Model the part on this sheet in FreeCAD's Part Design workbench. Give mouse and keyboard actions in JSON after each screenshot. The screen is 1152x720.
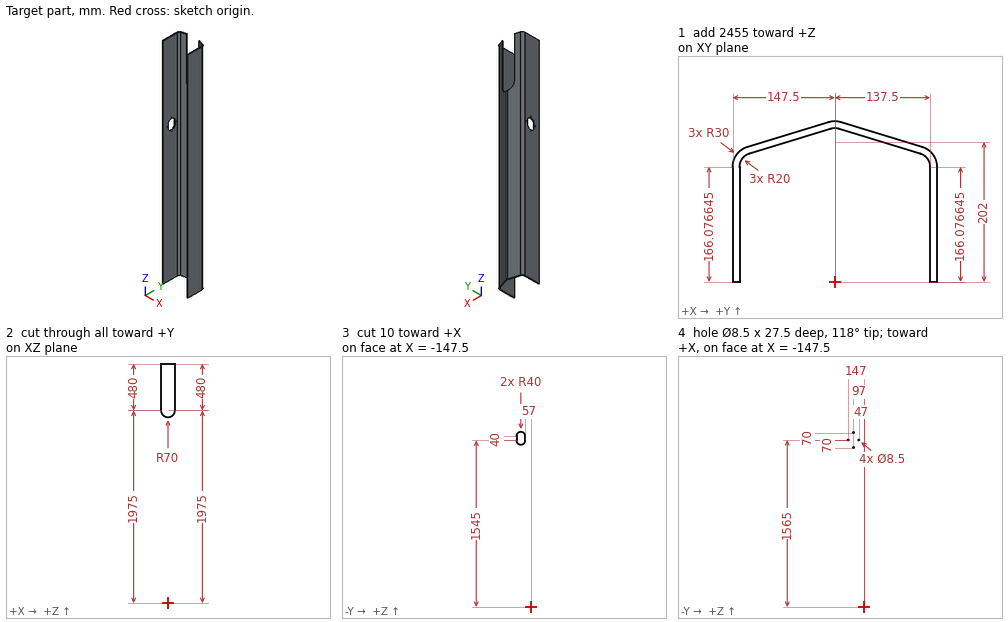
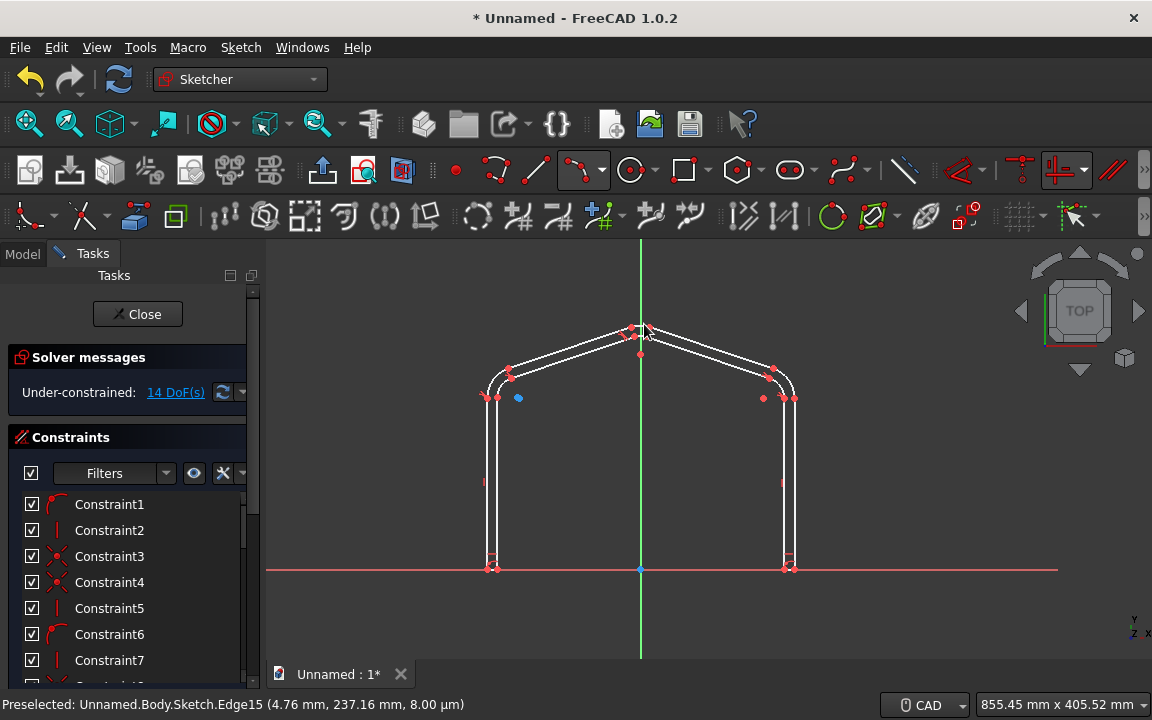
{"action": "scroll", "coordinate": [505, 382], "scroll_direction": "up", "scroll_amount": 3}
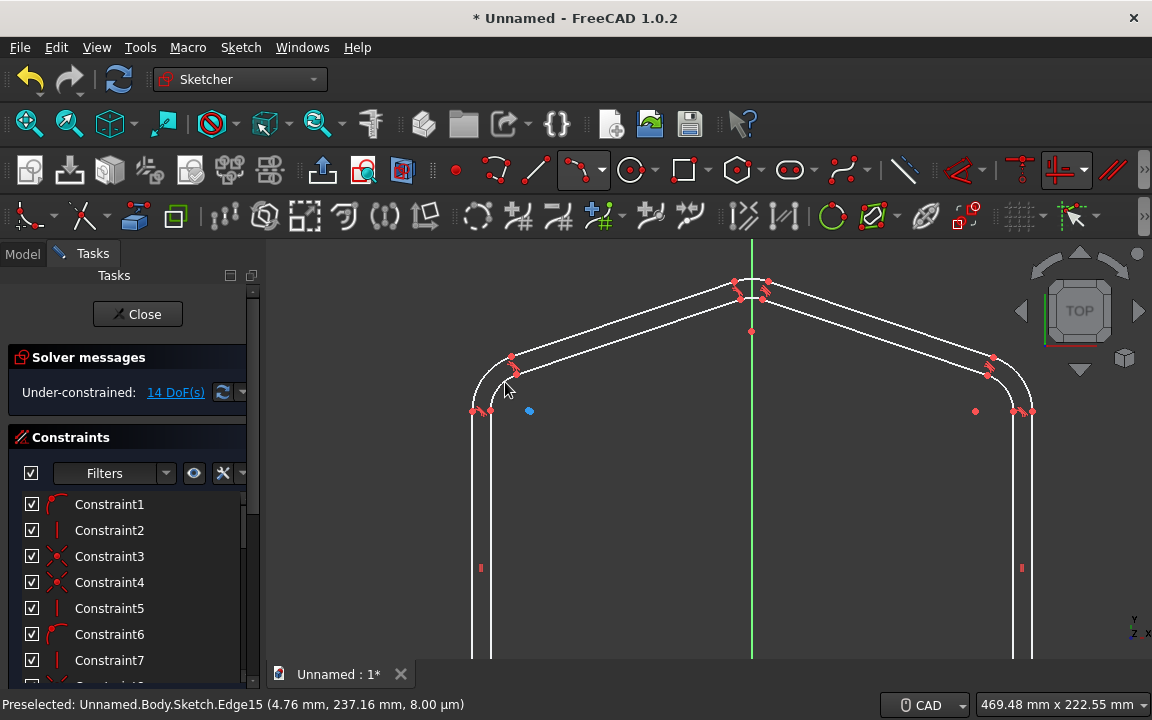
{"action": "left_click", "coordinate": [504, 382]}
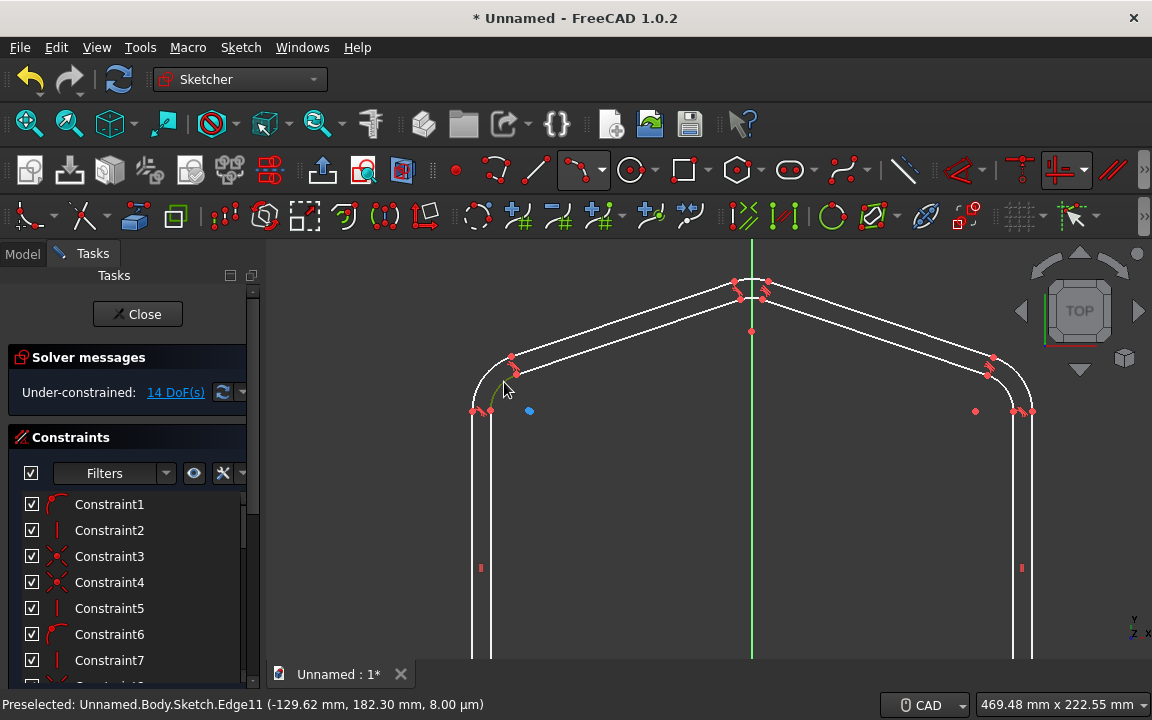
{"action": "left_click", "coordinate": [493, 367]}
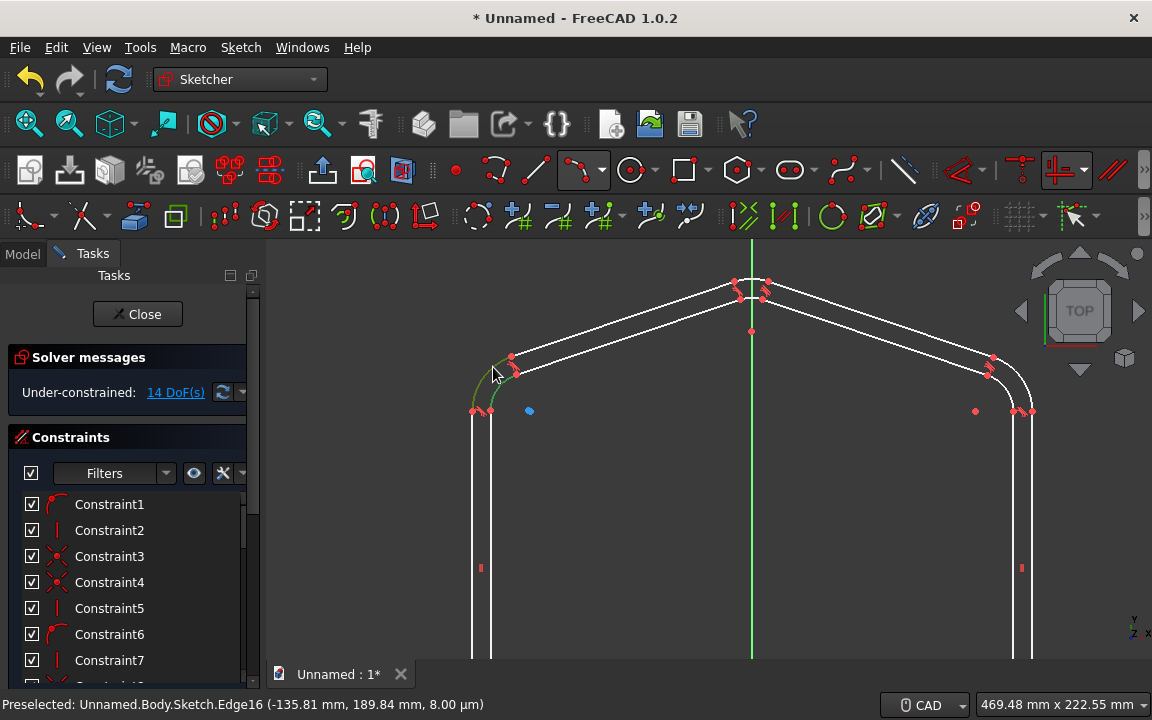
{"action": "left_click", "coordinate": [1020, 170]}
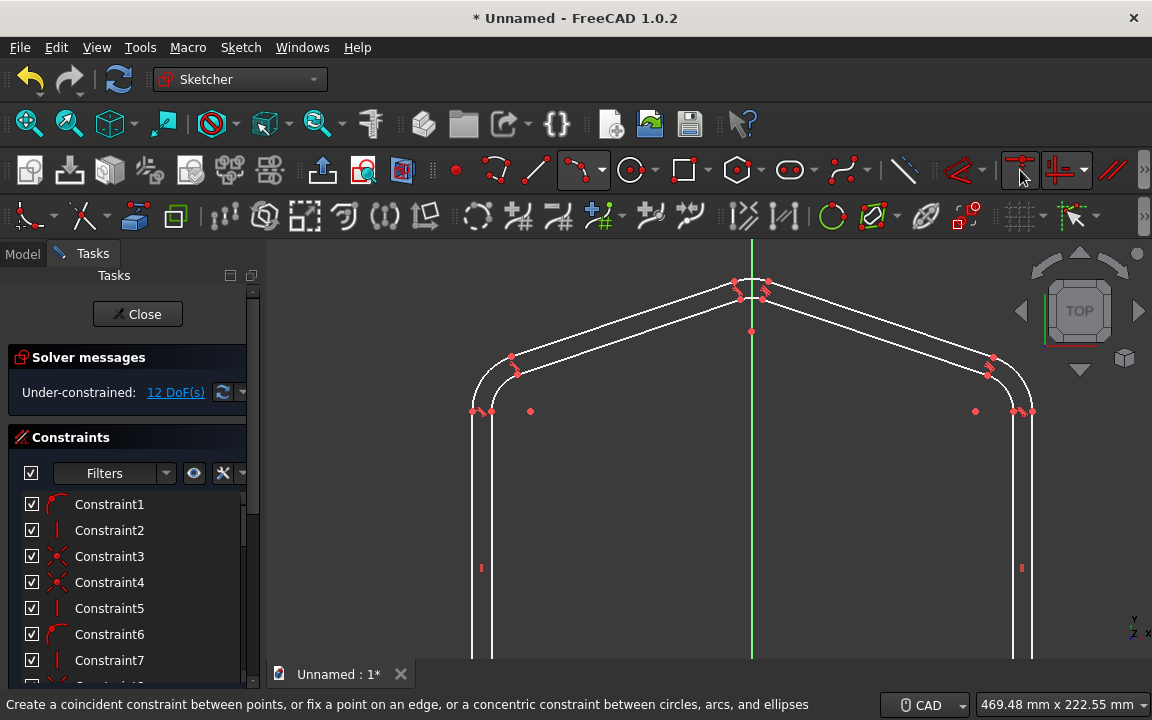
{"action": "left_click", "coordinate": [506, 382]}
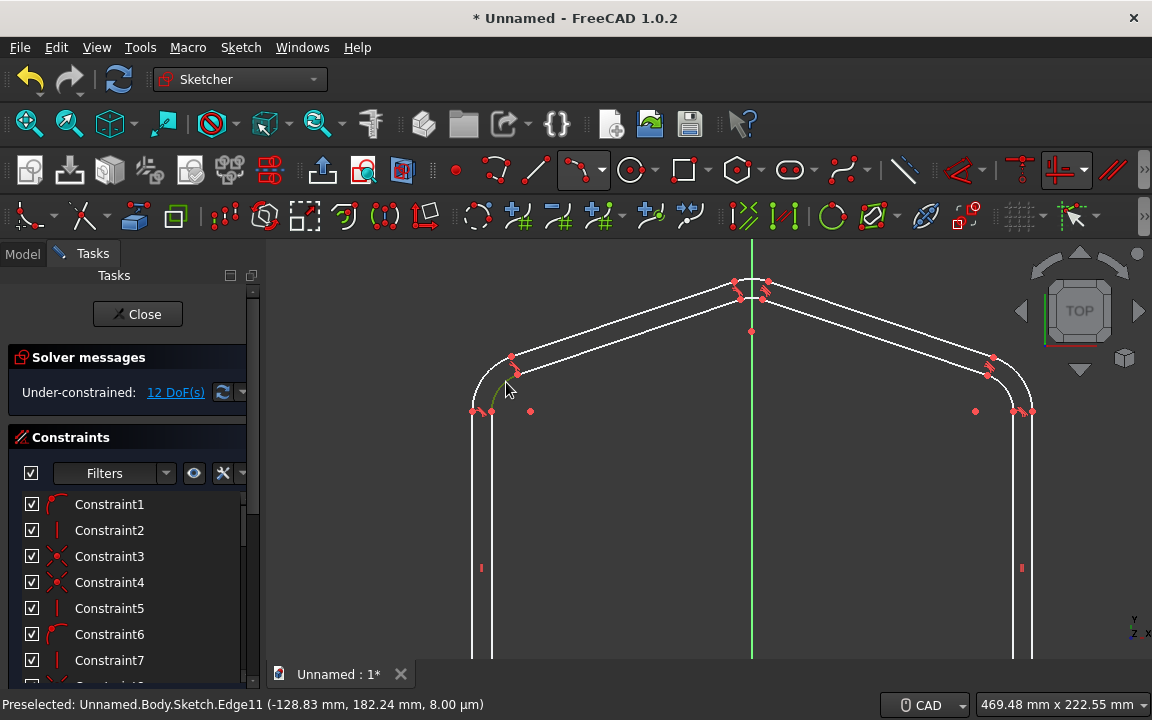
{"action": "scroll", "coordinate": [752, 298], "scroll_direction": "up", "scroll_amount": 2}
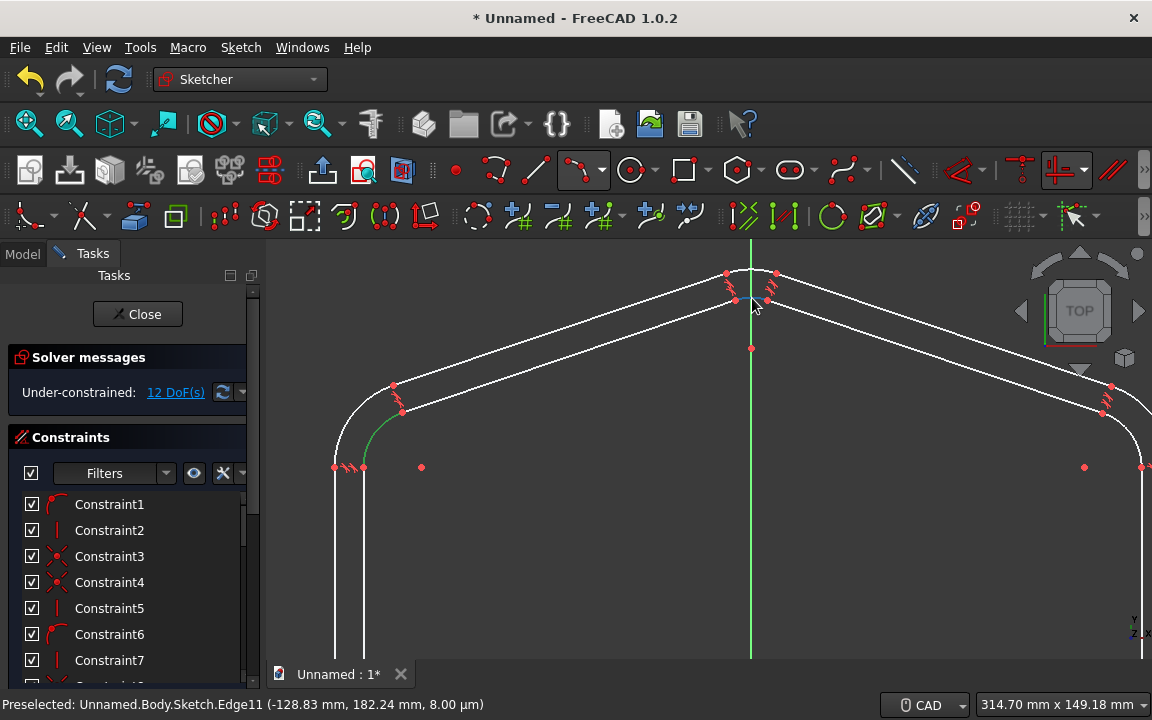
{"action": "left_click", "coordinate": [751, 298]}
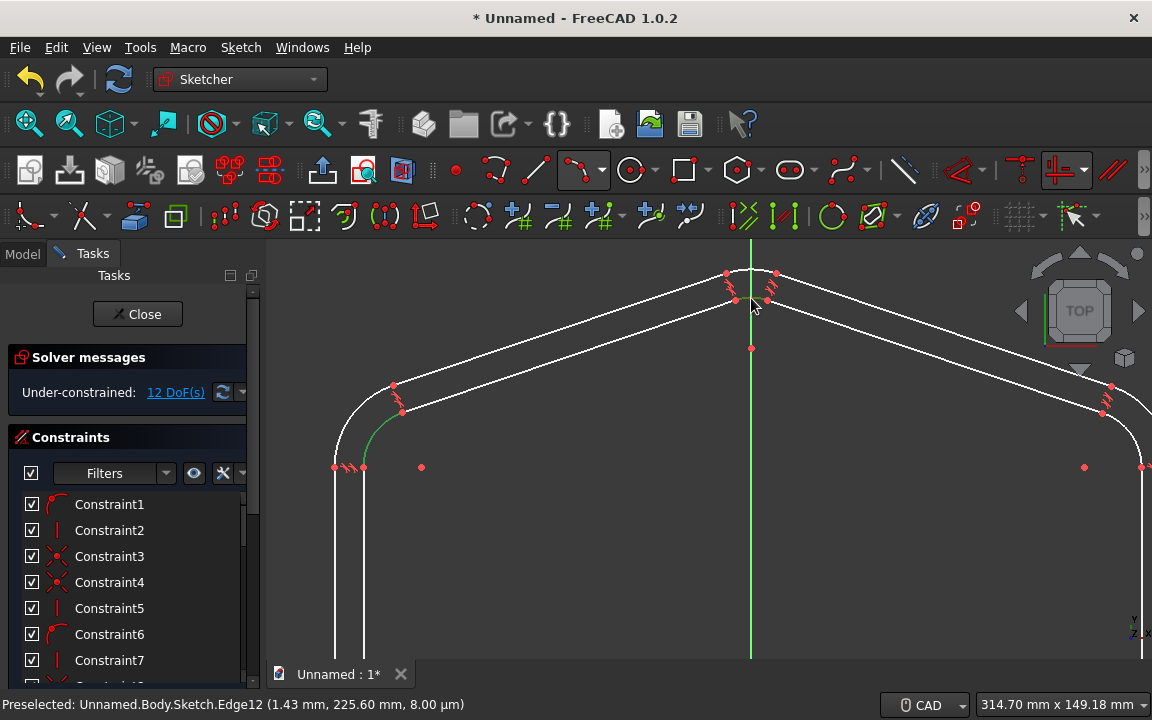
{"action": "scroll", "coordinate": [576, 357], "scroll_direction": "down", "scroll_amount": 5}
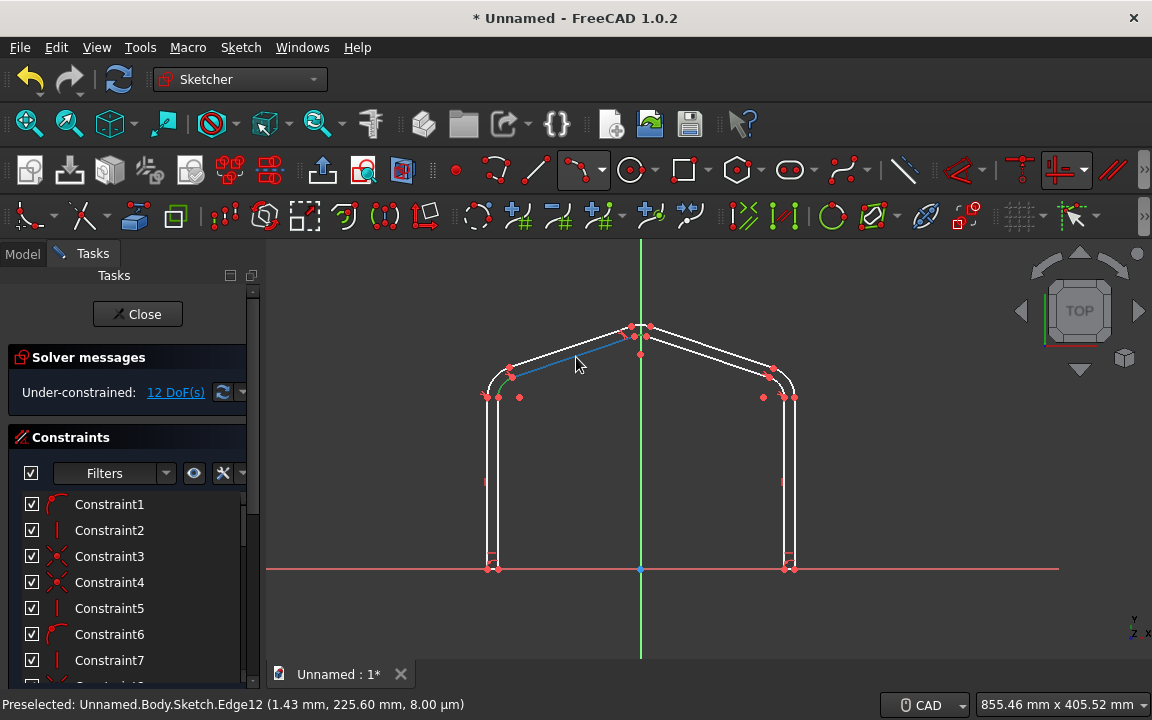
{"action": "scroll", "coordinate": [783, 390], "scroll_direction": "up", "scroll_amount": 3}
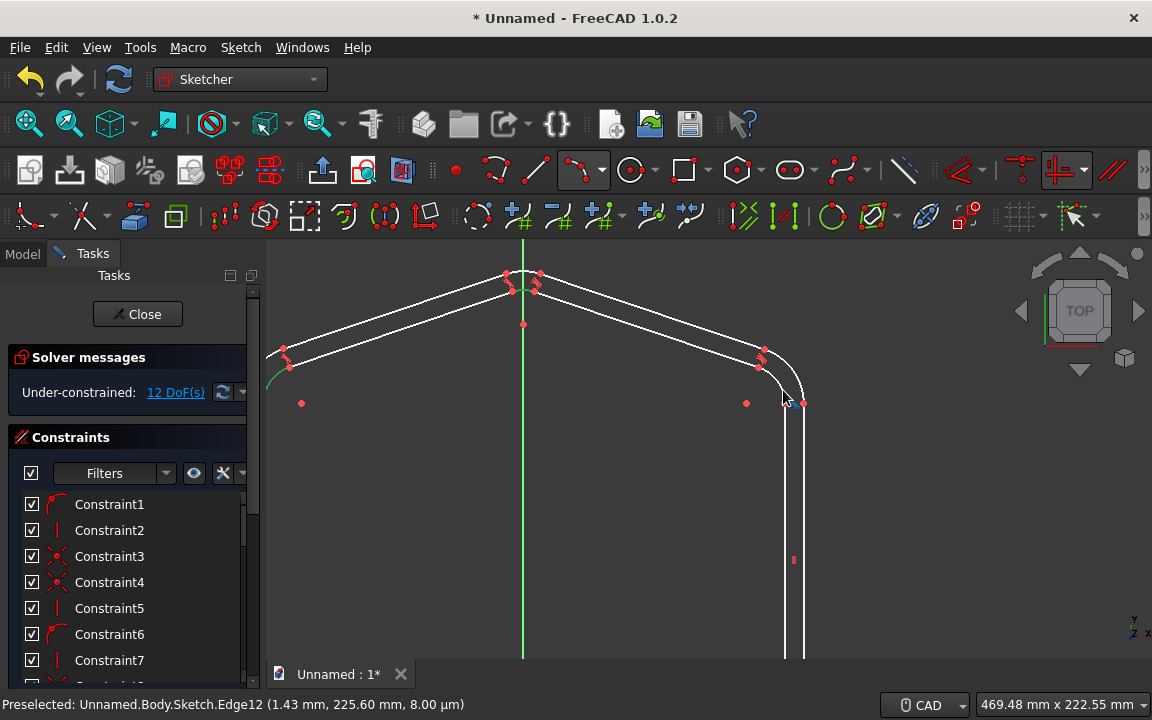
{"action": "left_click", "coordinate": [782, 390]}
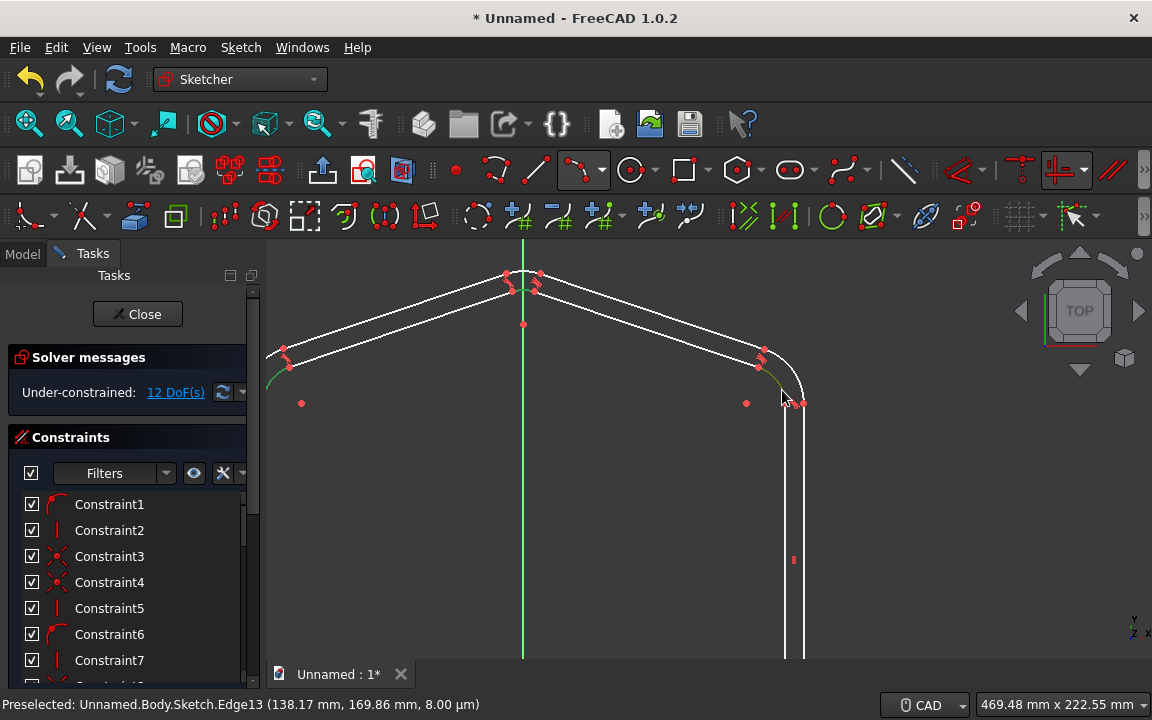
{"action": "key", "text": "e"}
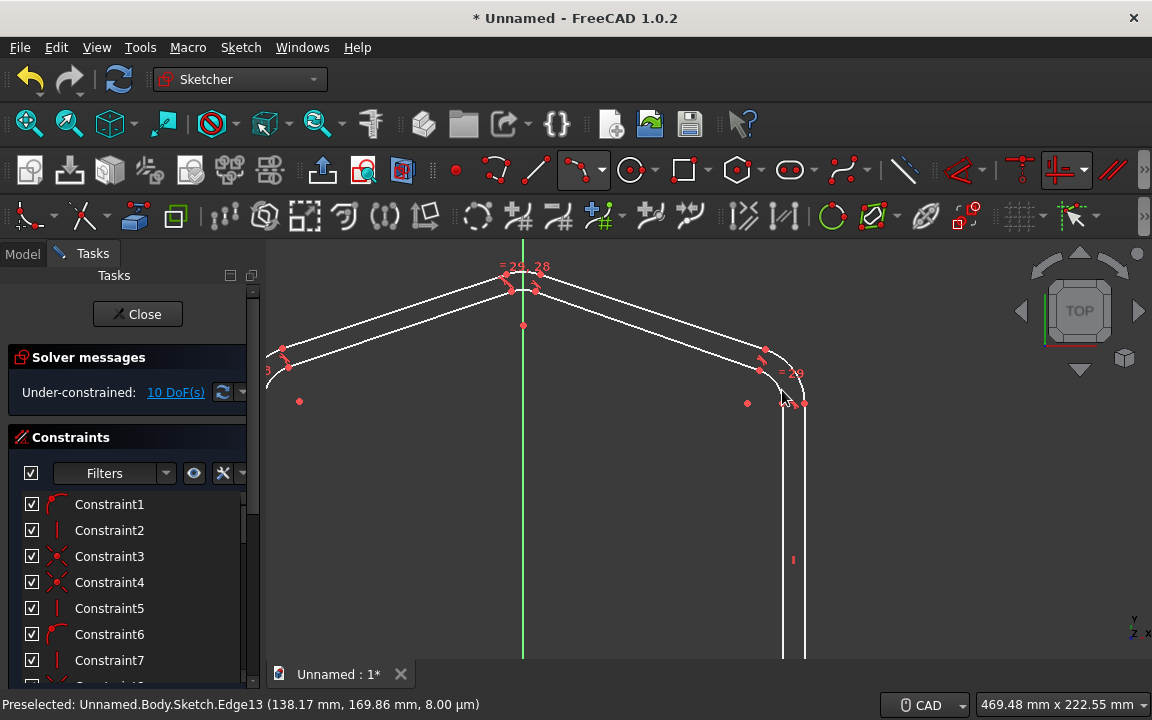
{"action": "left_click", "coordinate": [801, 383]}